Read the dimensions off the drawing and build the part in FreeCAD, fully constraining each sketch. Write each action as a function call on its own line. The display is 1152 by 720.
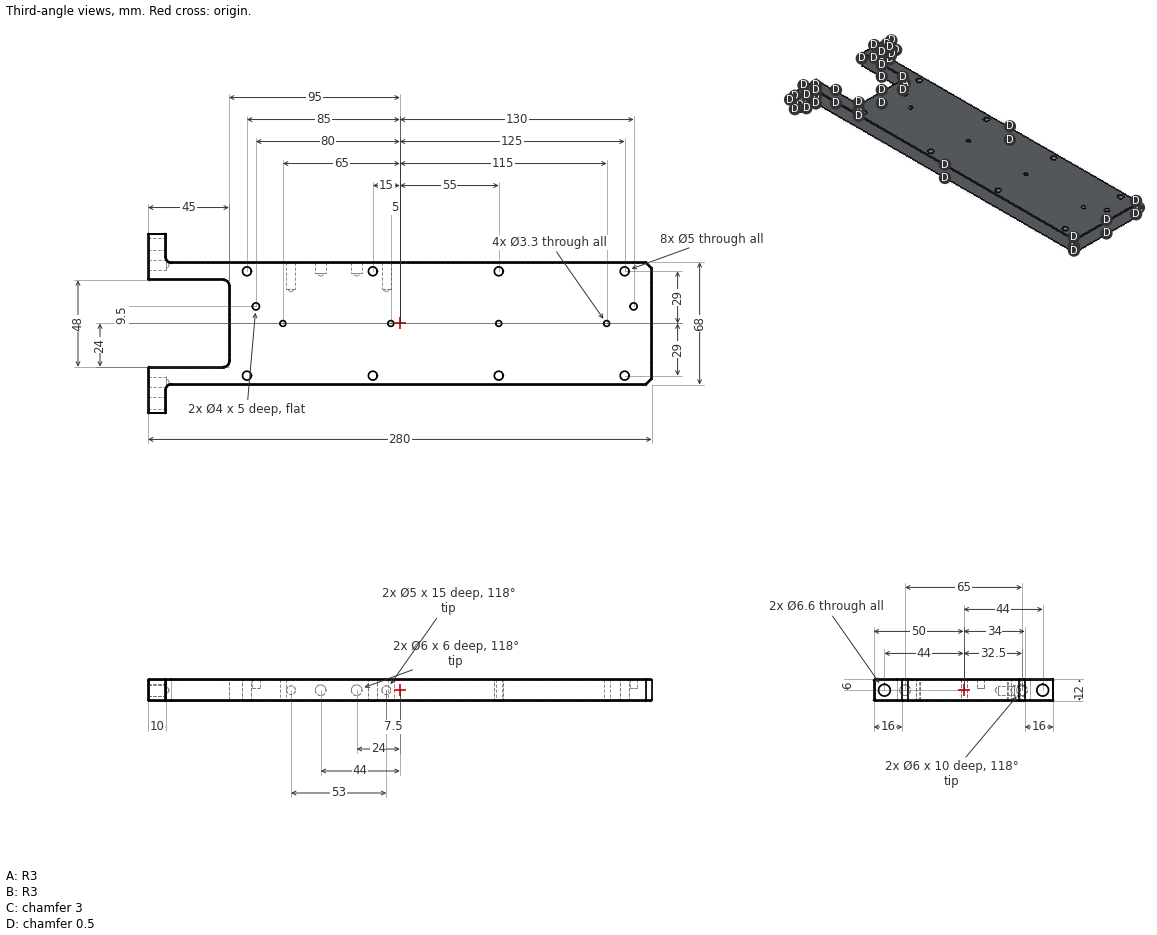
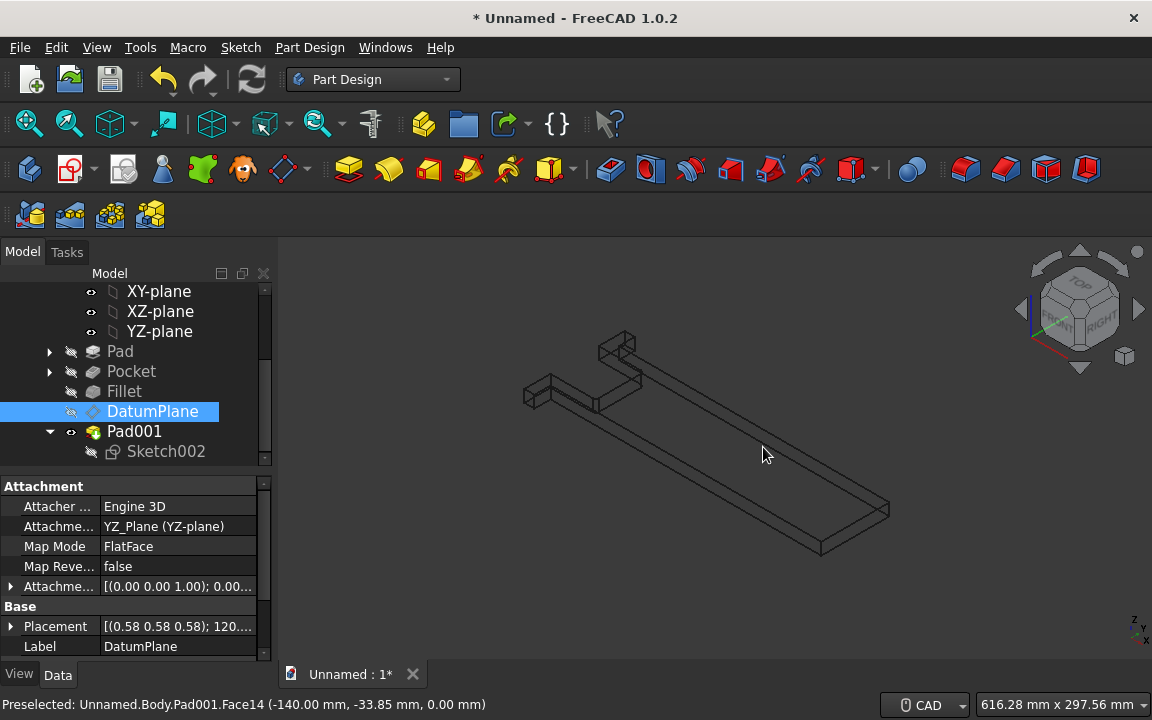
click(551, 393)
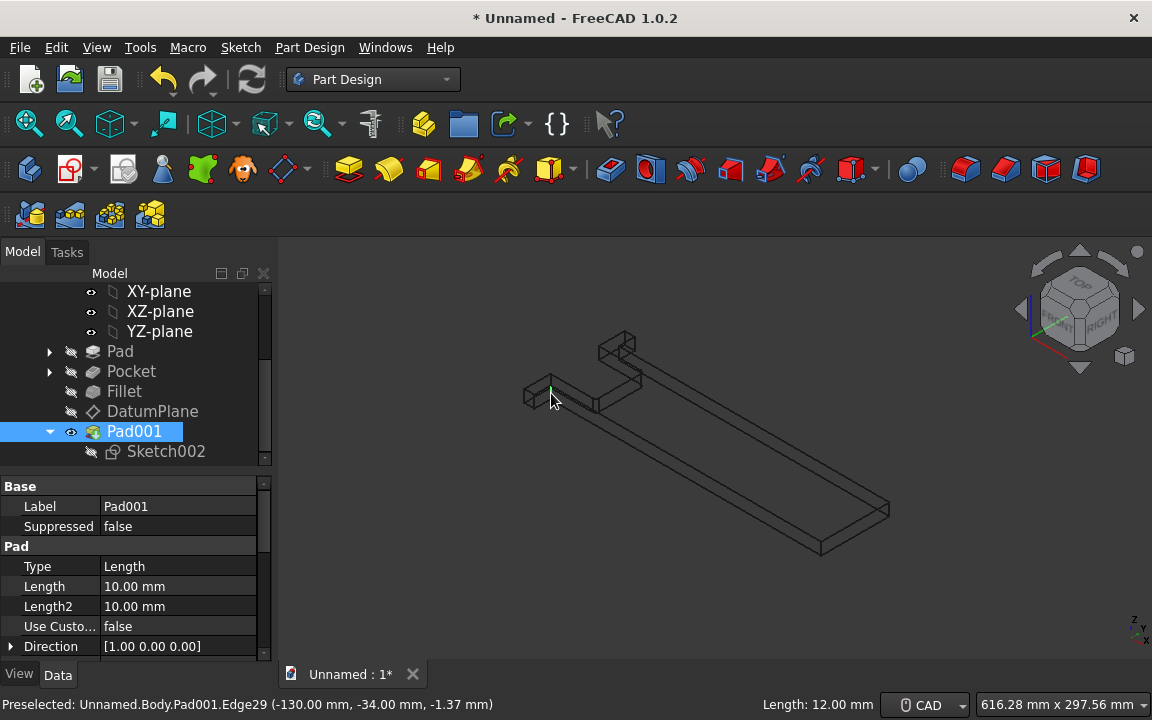
scroll(619, 352, up, 6)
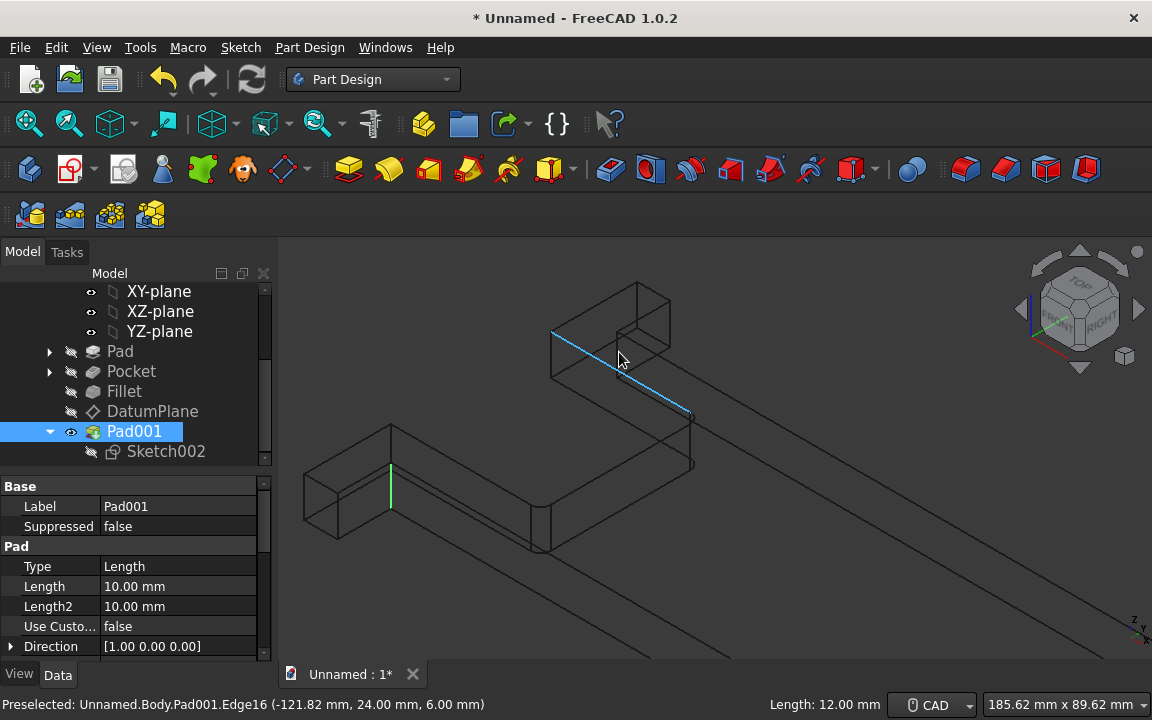
click(617, 354, ctrl)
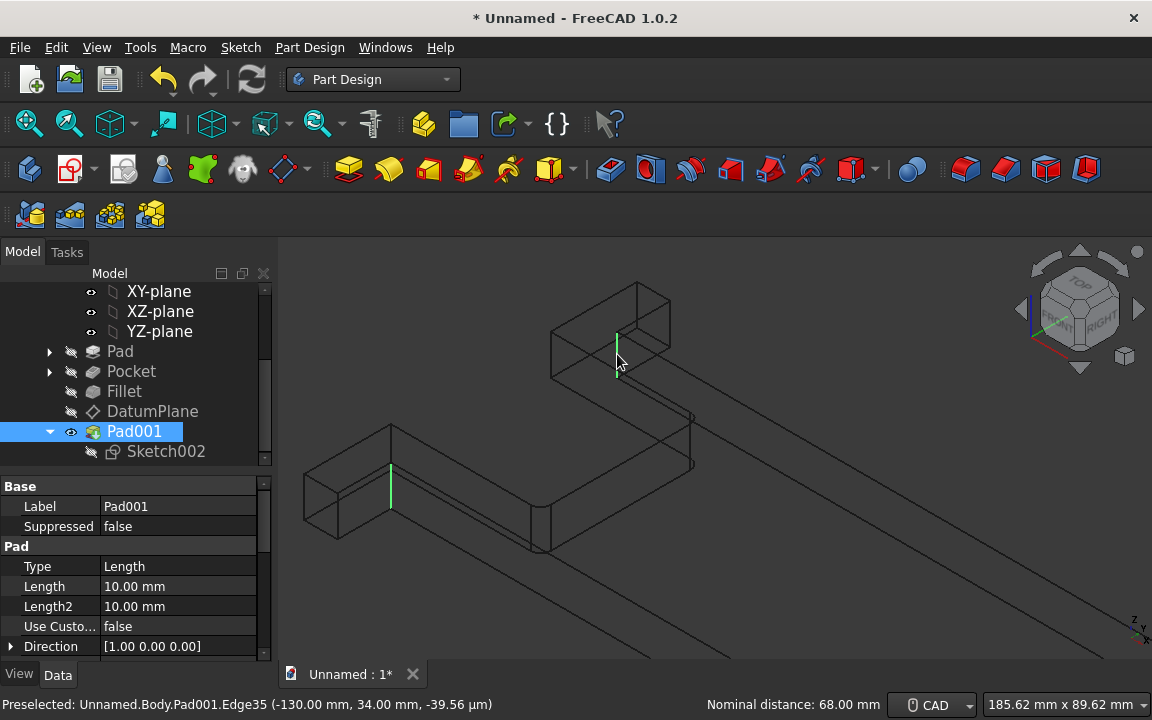
key(v)
key(1)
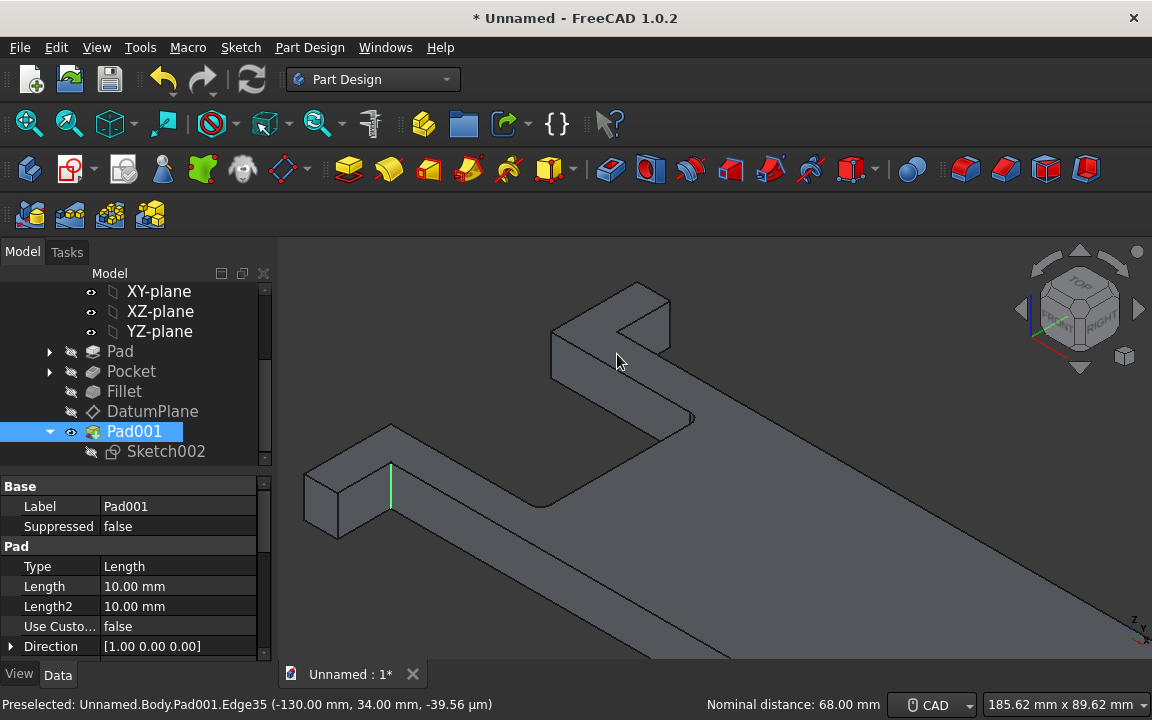
click(966, 170)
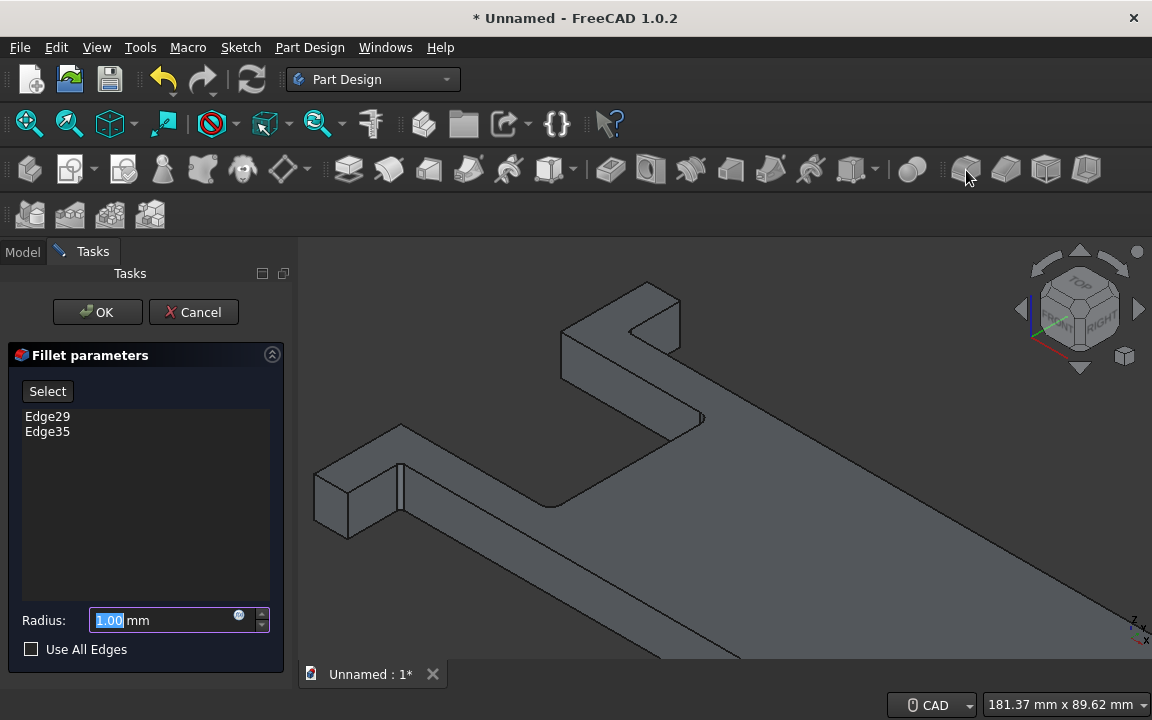
text(3)
key(Tab)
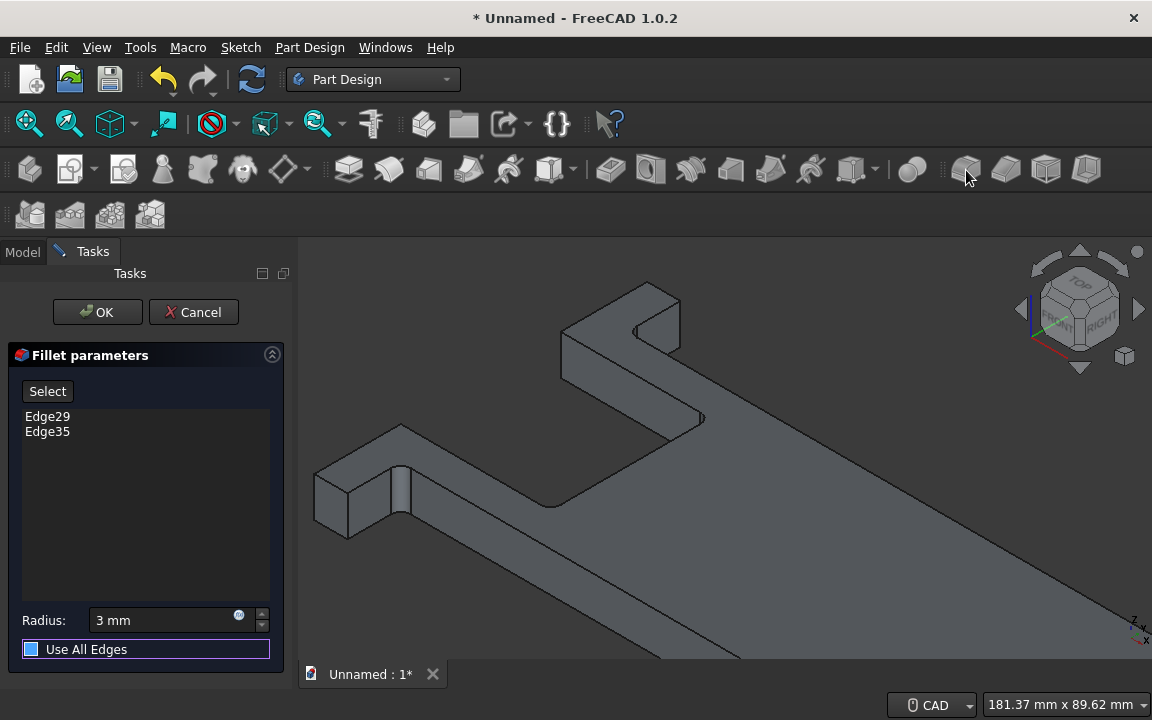
click(98, 312)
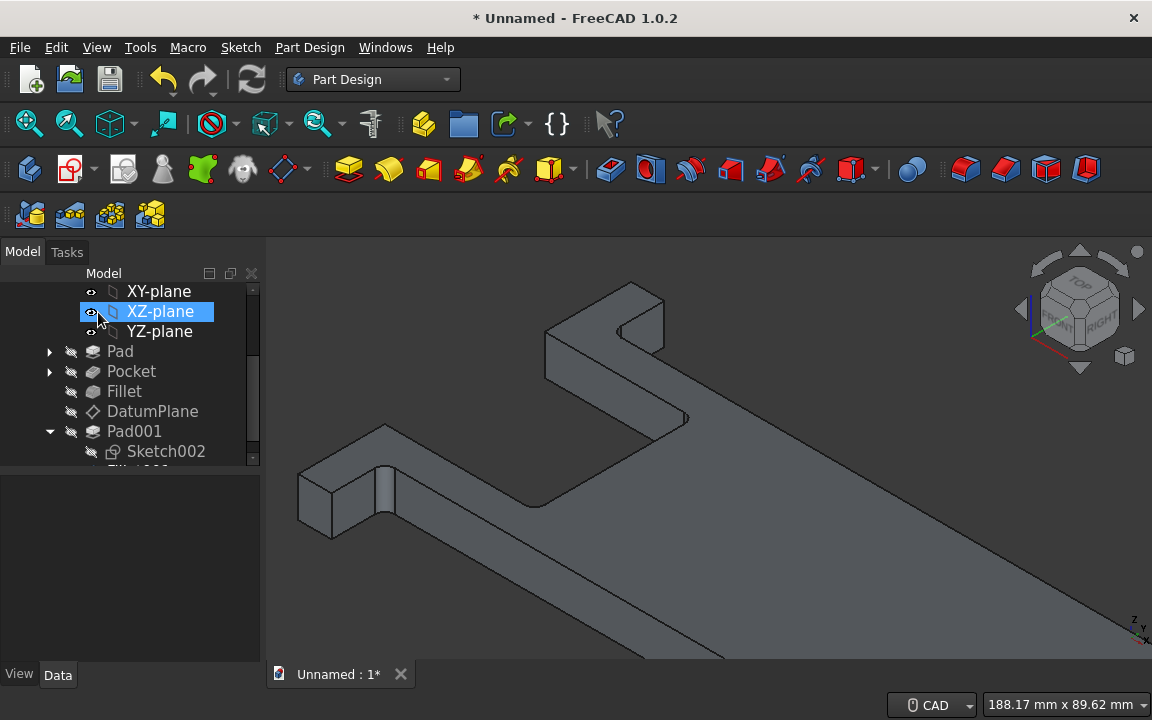
click(30, 124)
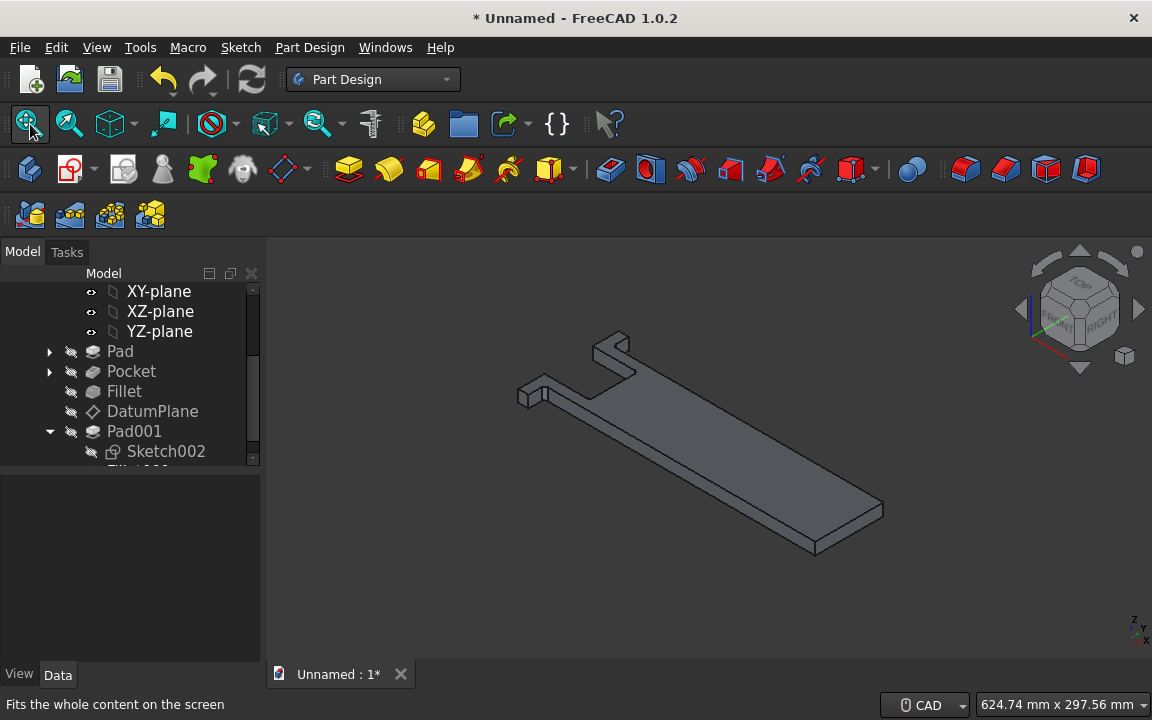
key(3)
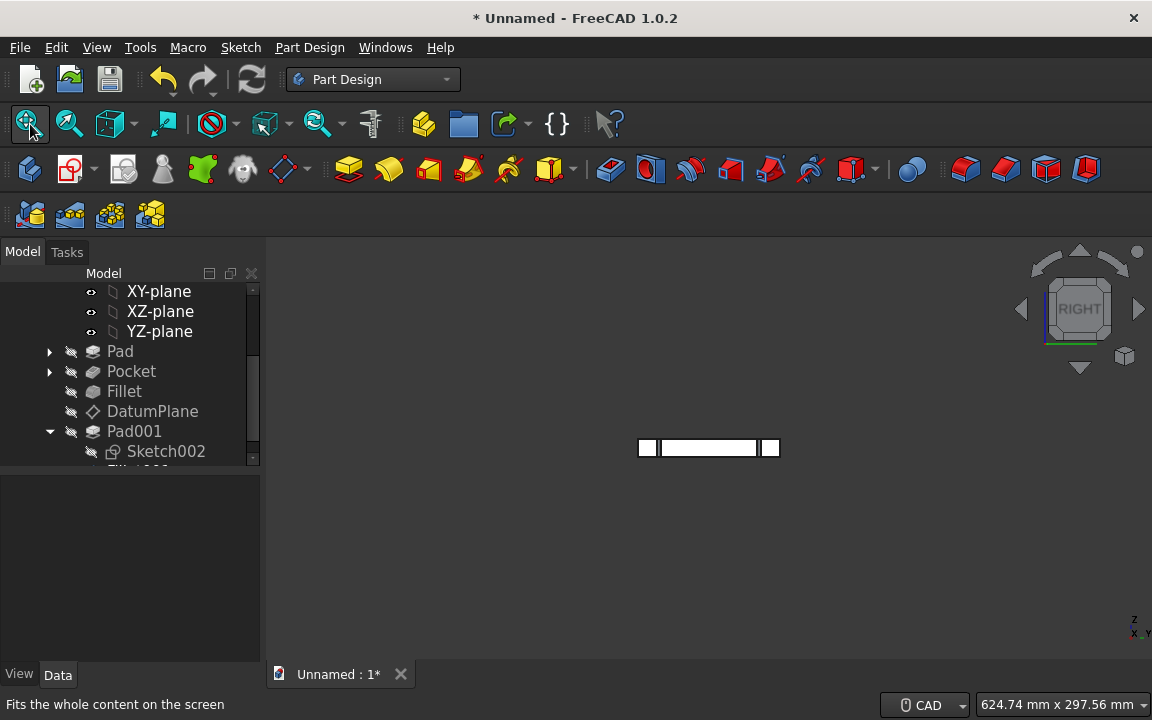
click(30, 124)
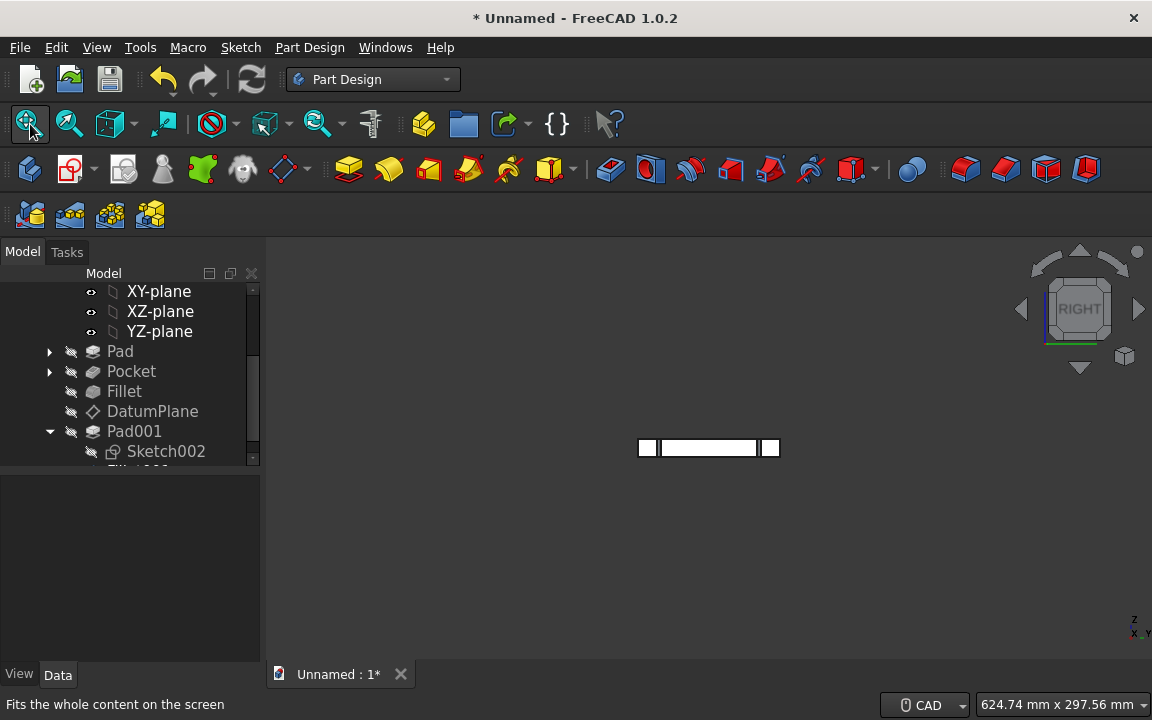
click(771, 447)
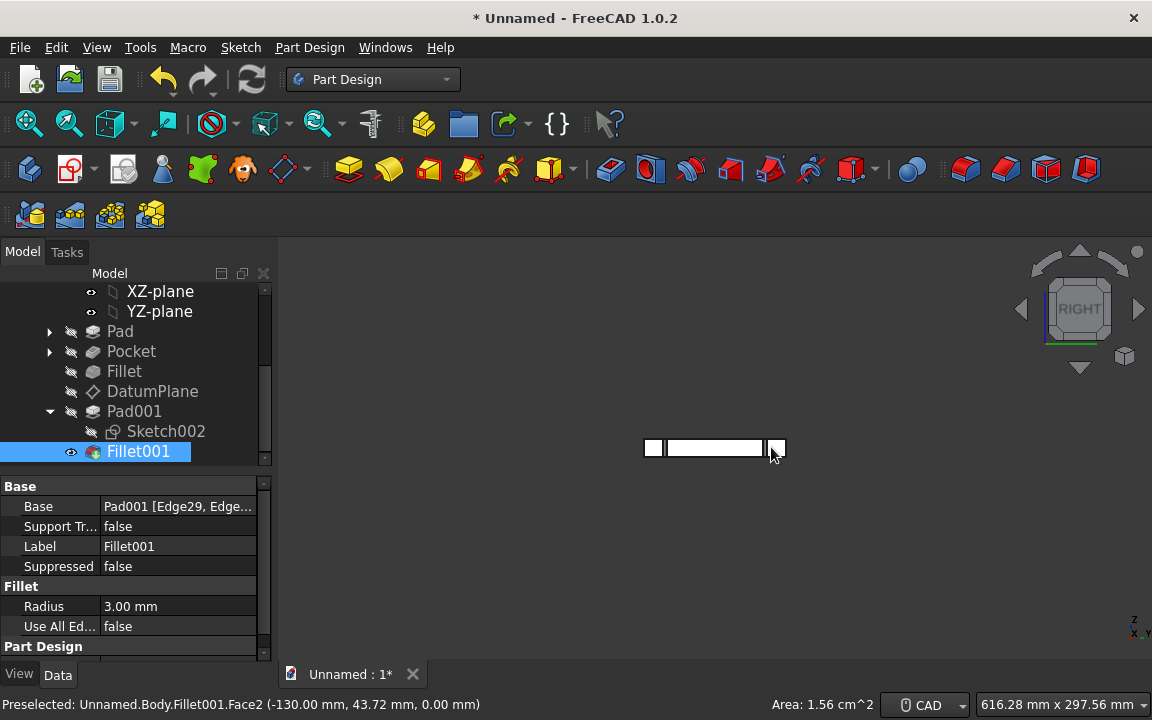
click(70, 170)